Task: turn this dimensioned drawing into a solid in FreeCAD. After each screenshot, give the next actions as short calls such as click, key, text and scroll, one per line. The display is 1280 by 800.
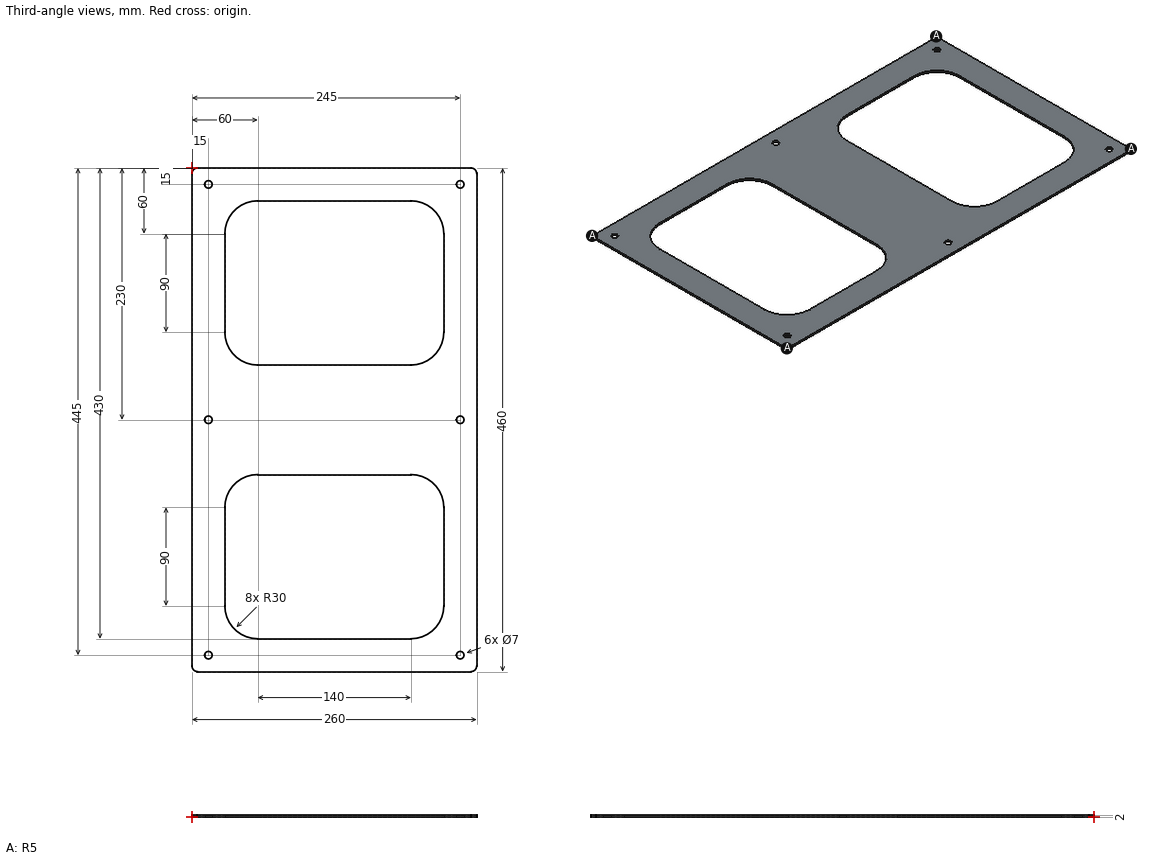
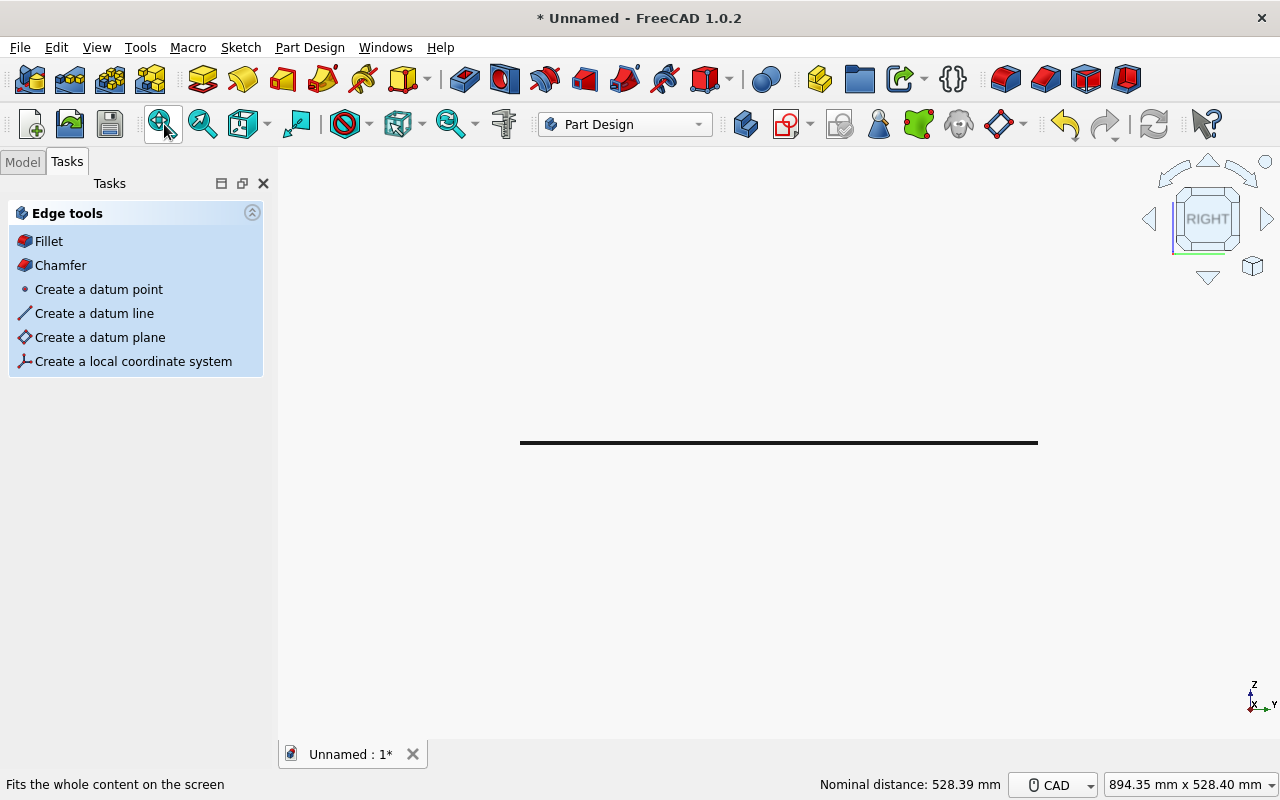
key(5)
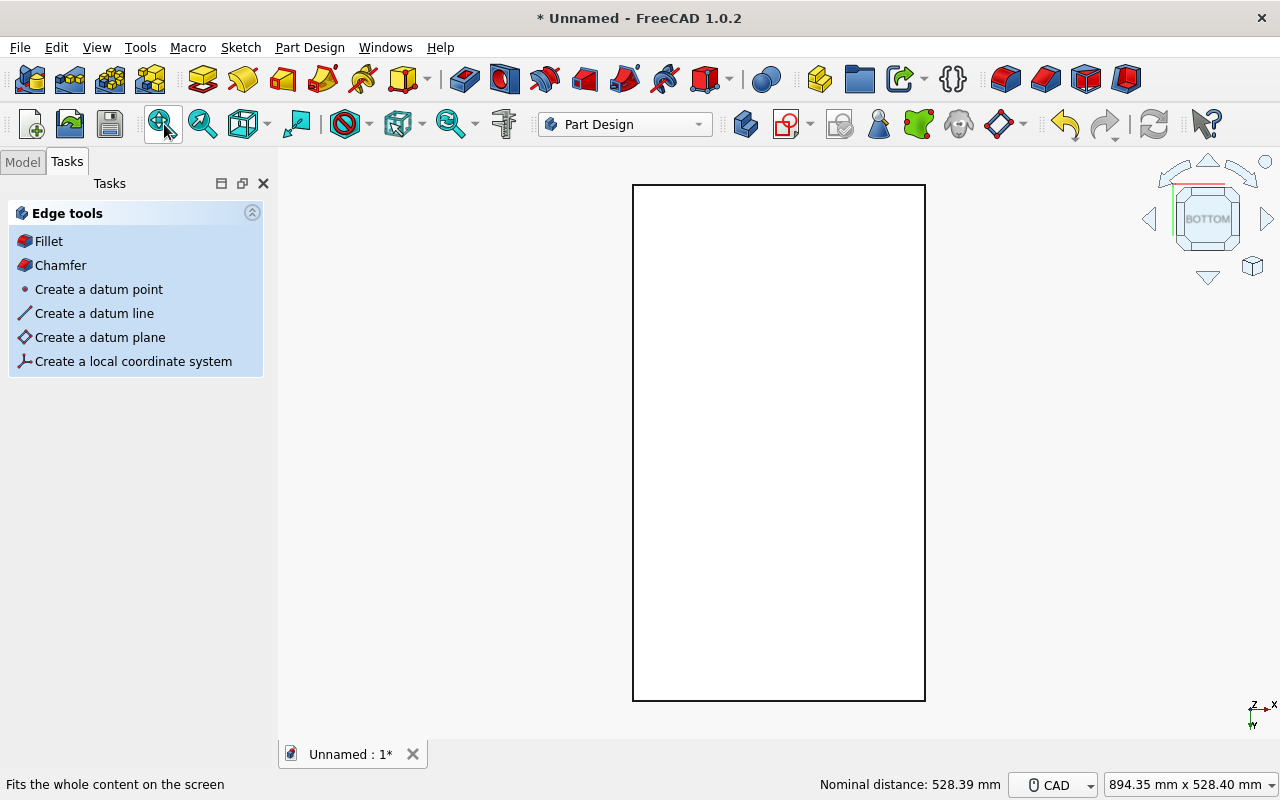
scroll(633, 700, up, 15)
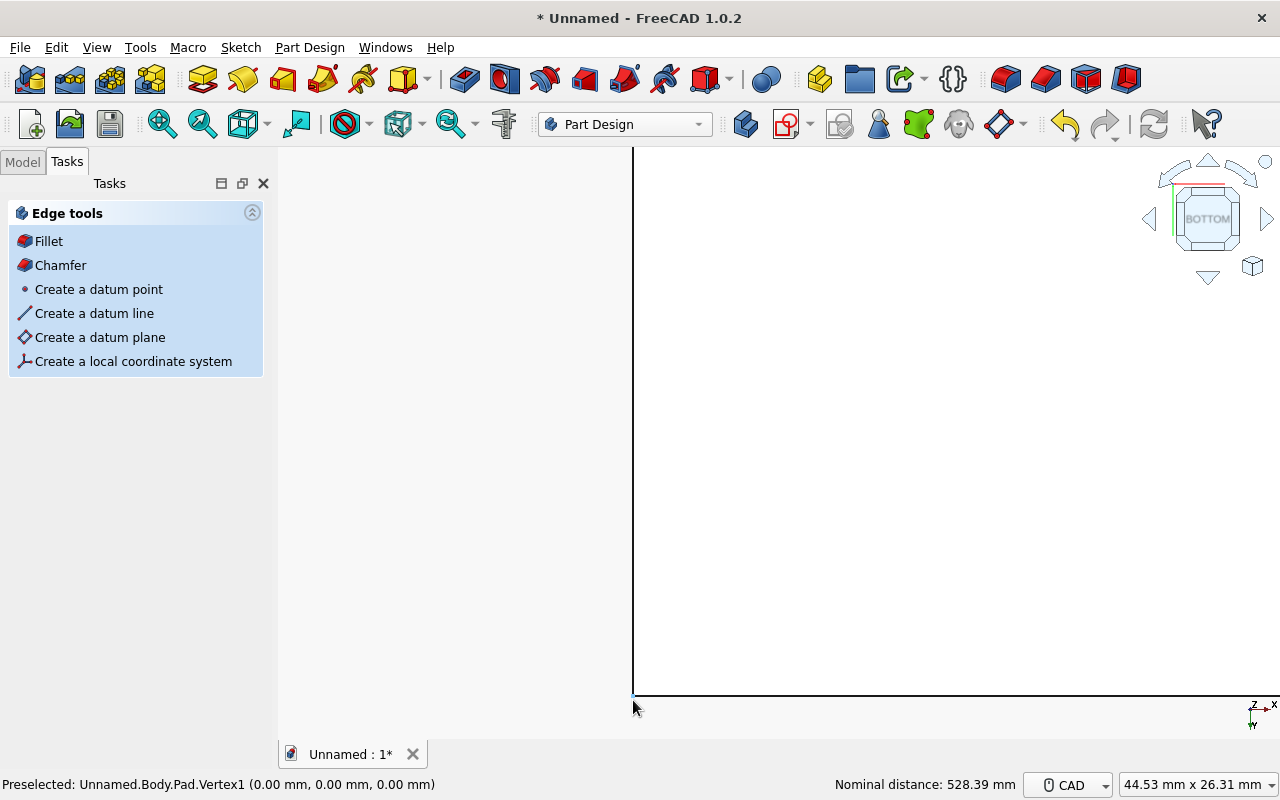
click(164, 124)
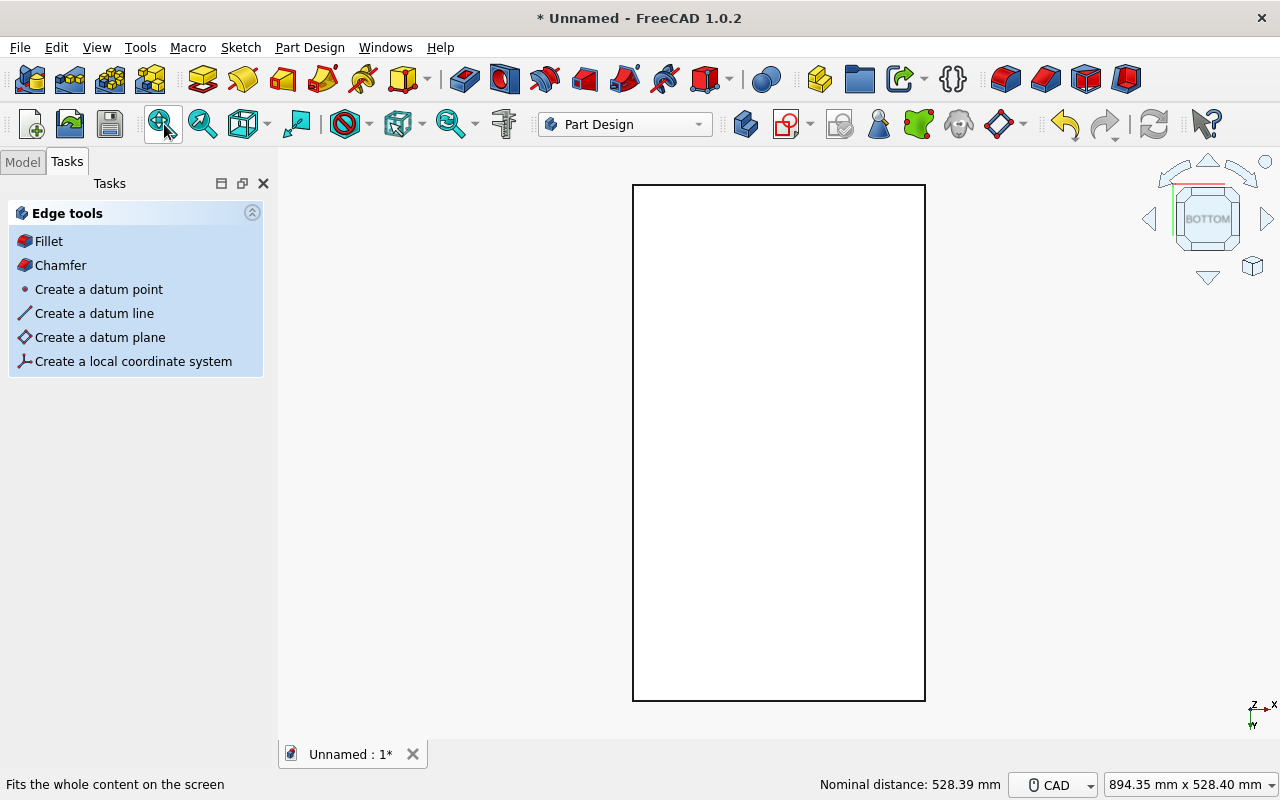
key(4)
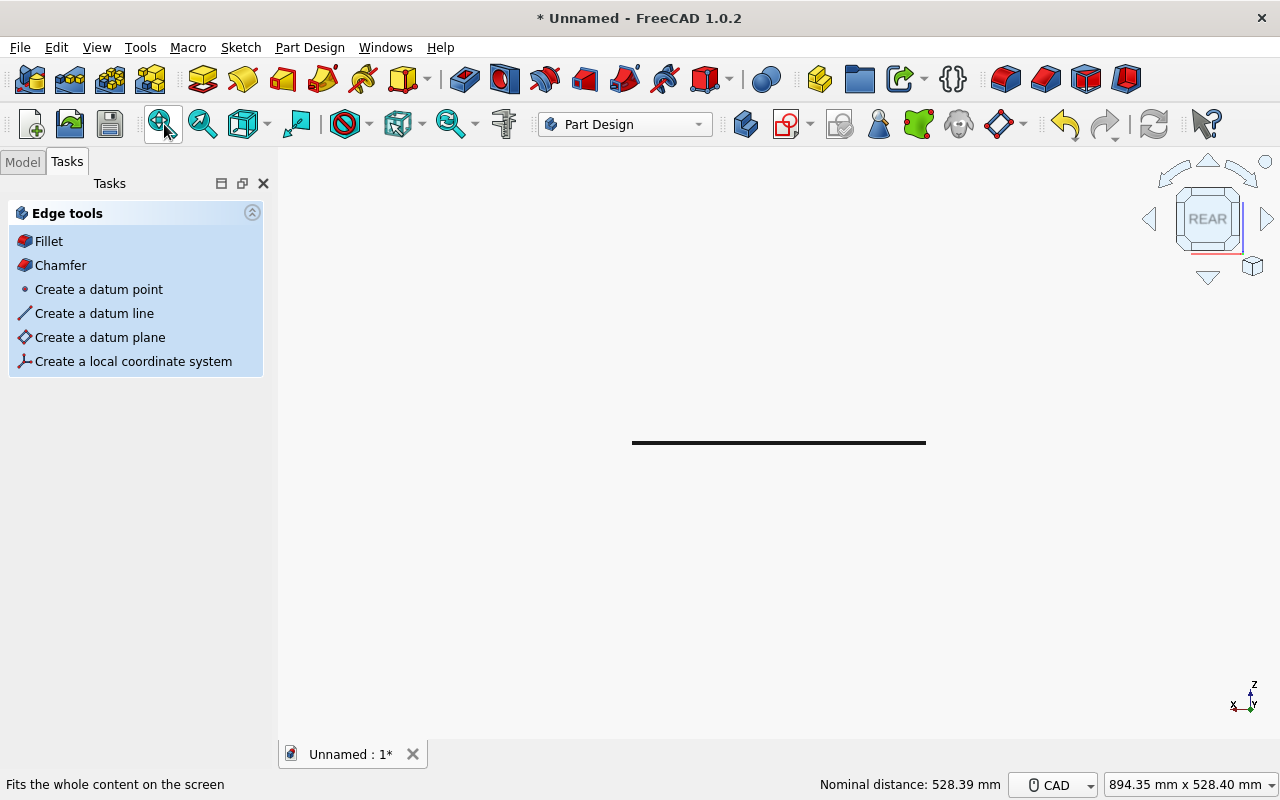
click(164, 124)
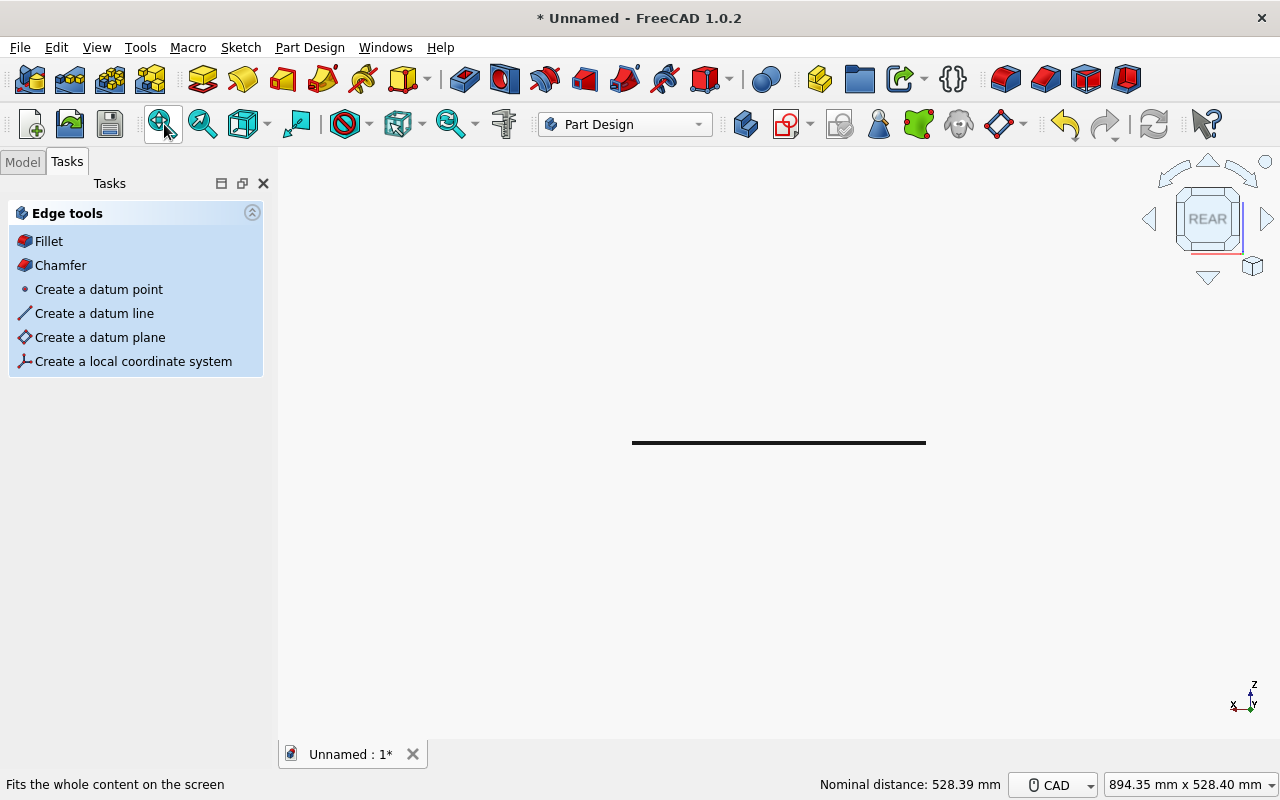
scroll(925, 442, up, 15)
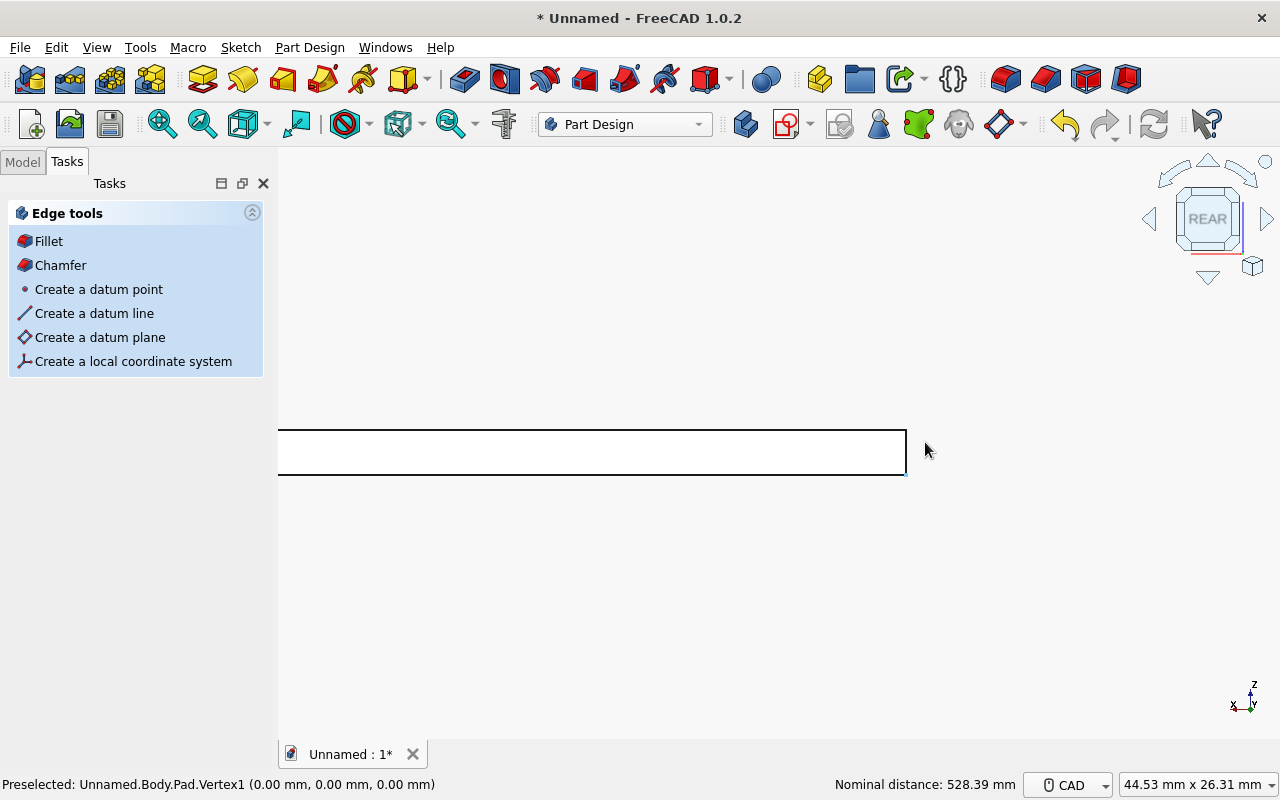
click(906, 452, ctrl)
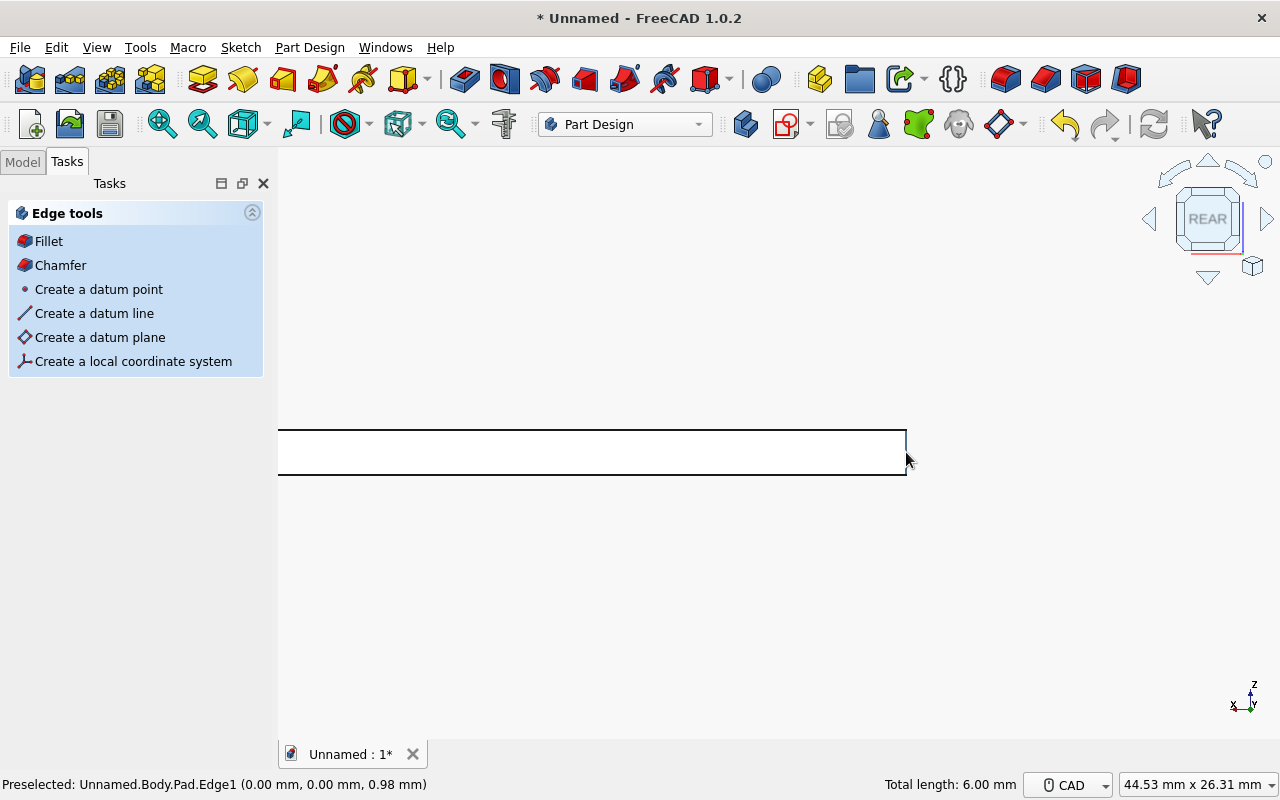
click(164, 124)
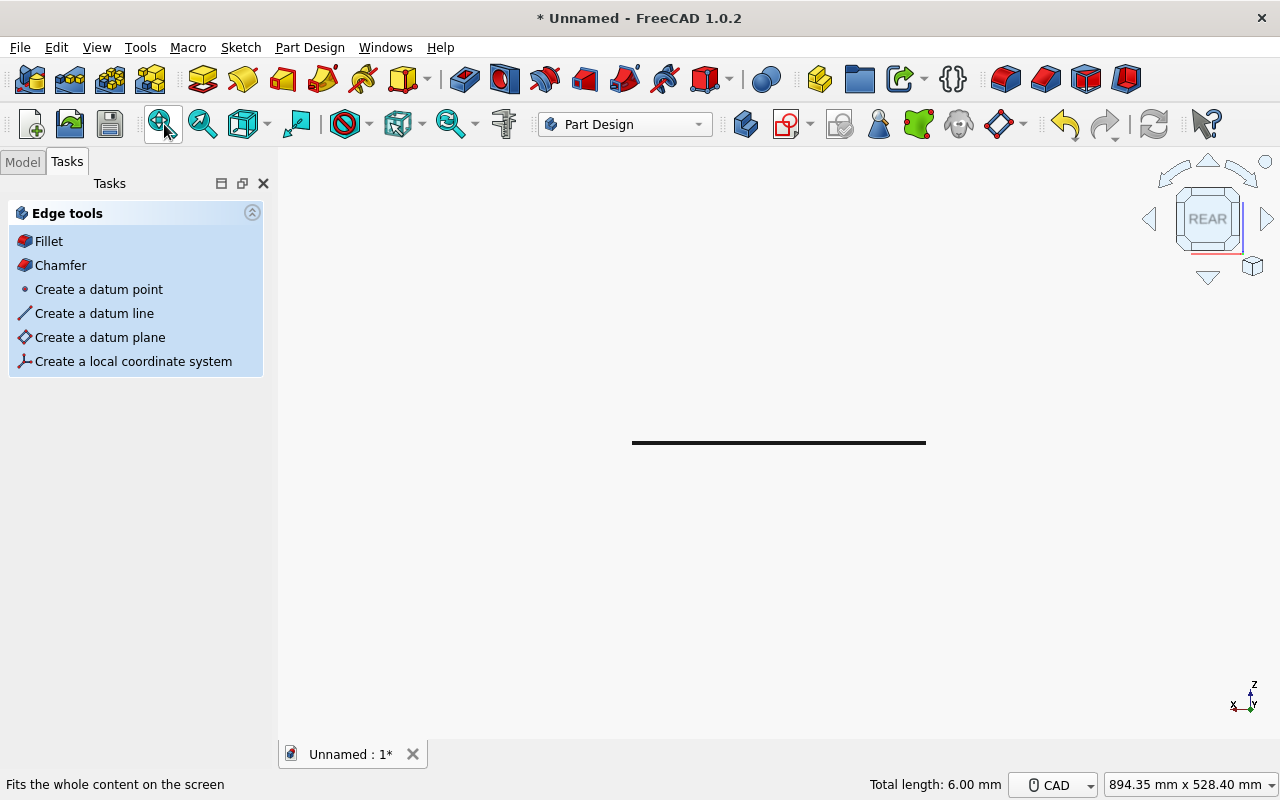
key(6)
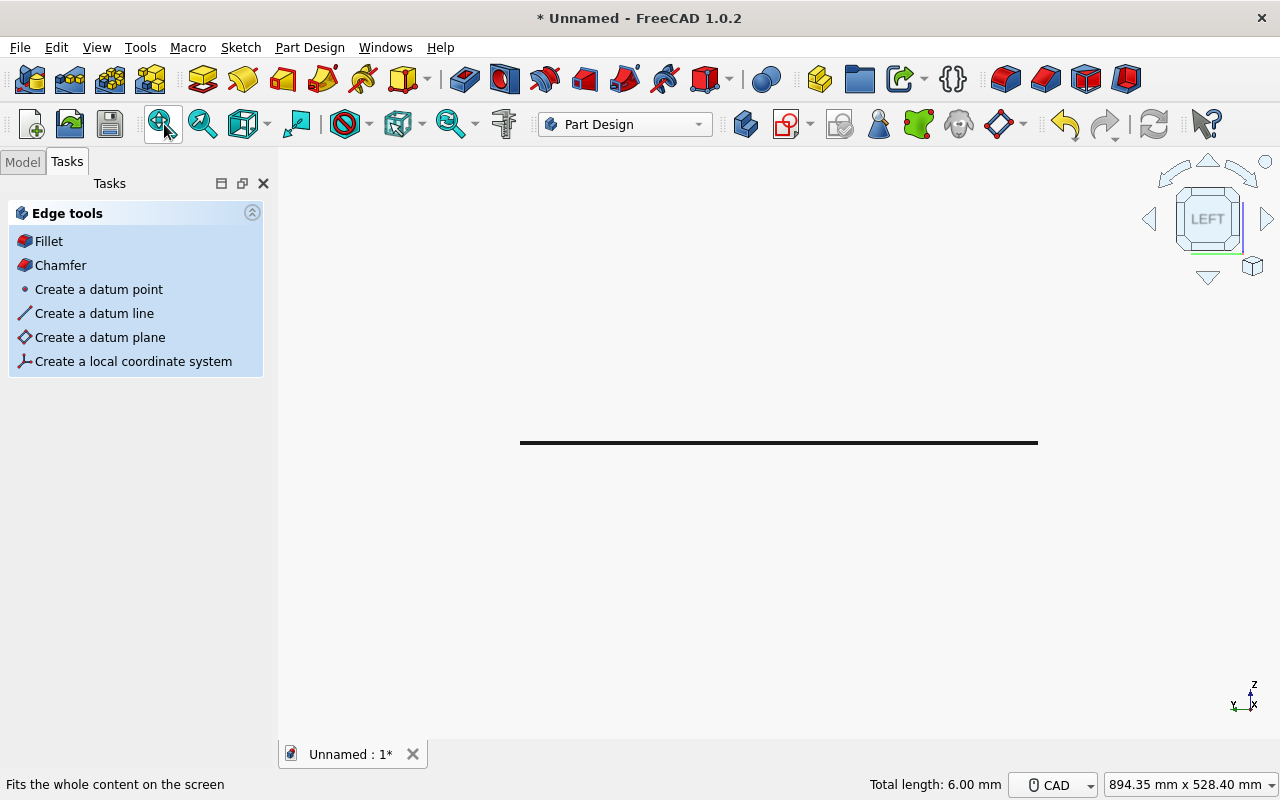
scroll(1037, 442, up, 15)